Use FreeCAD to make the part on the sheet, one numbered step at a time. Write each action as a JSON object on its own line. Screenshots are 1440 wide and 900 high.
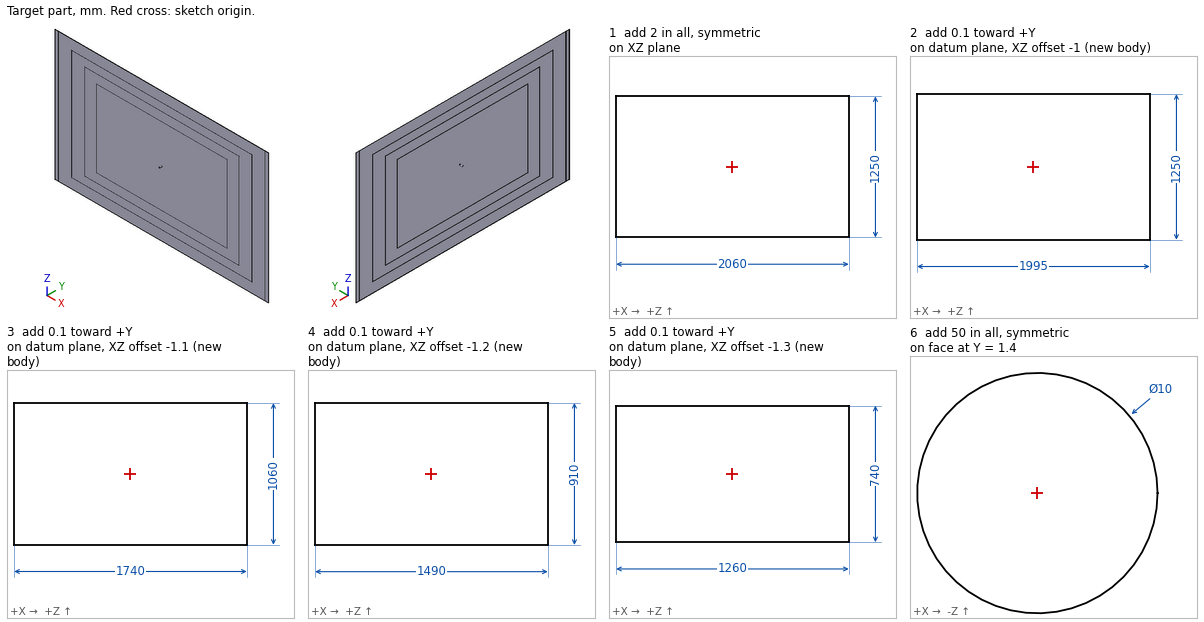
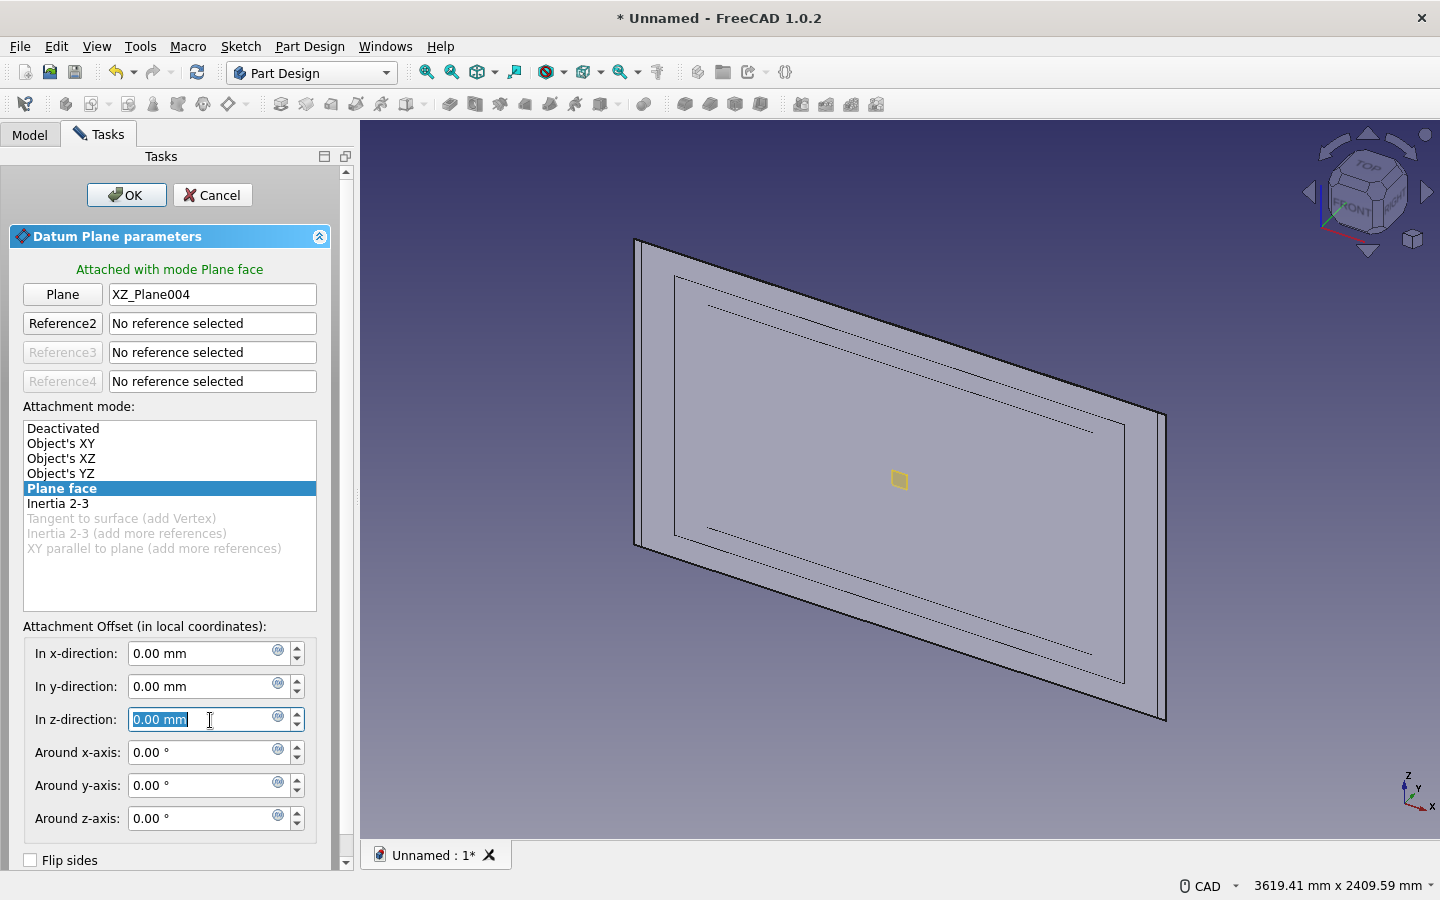
{"action": "type", "text": "-1.3"}
{"action": "key", "text": "Tab"}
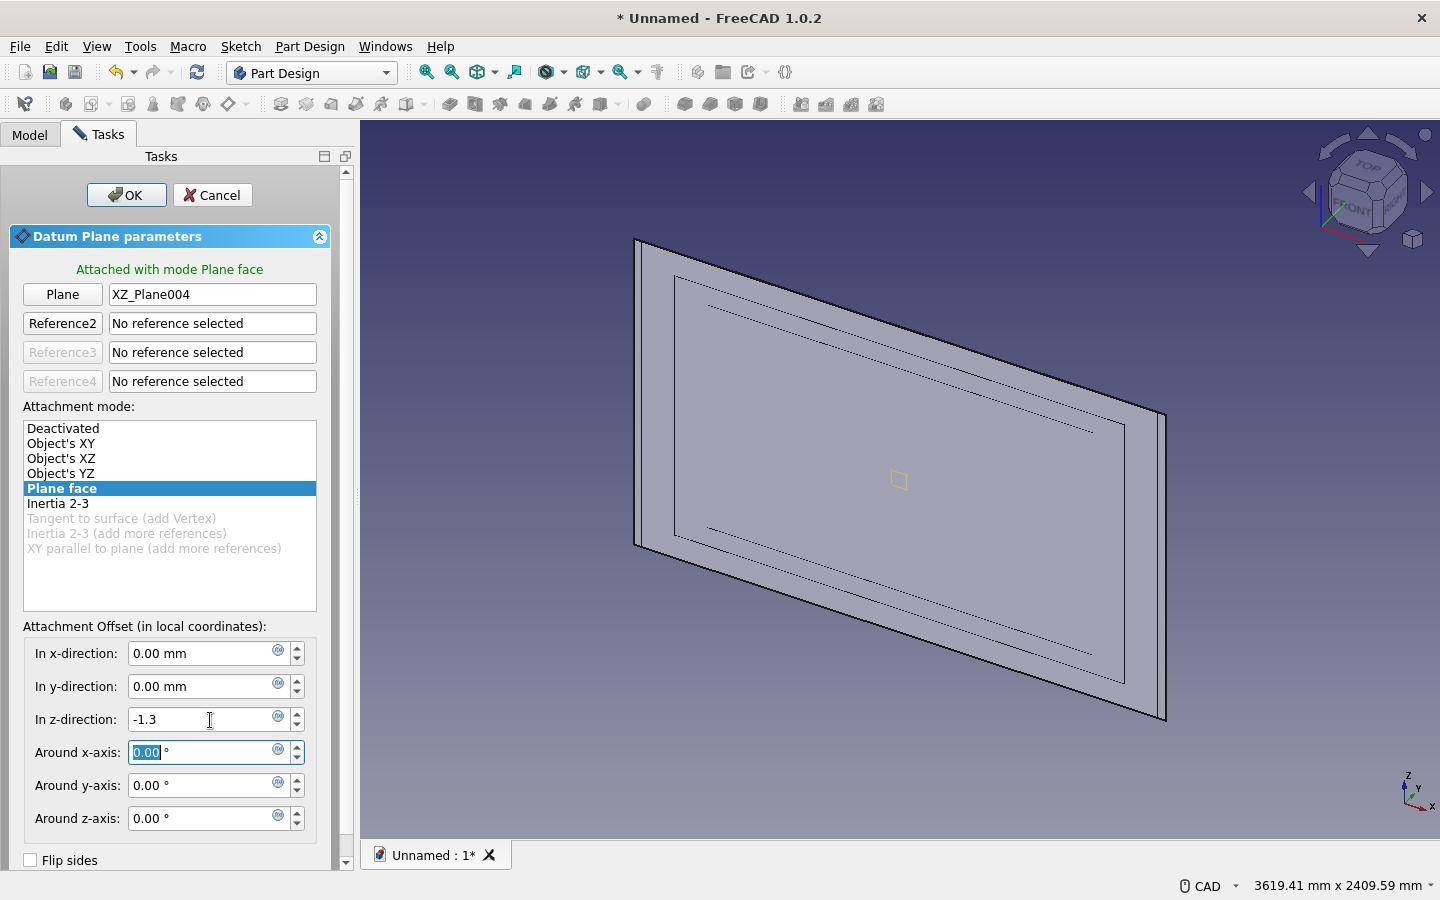
{"action": "left_click", "coordinate": [127, 195]}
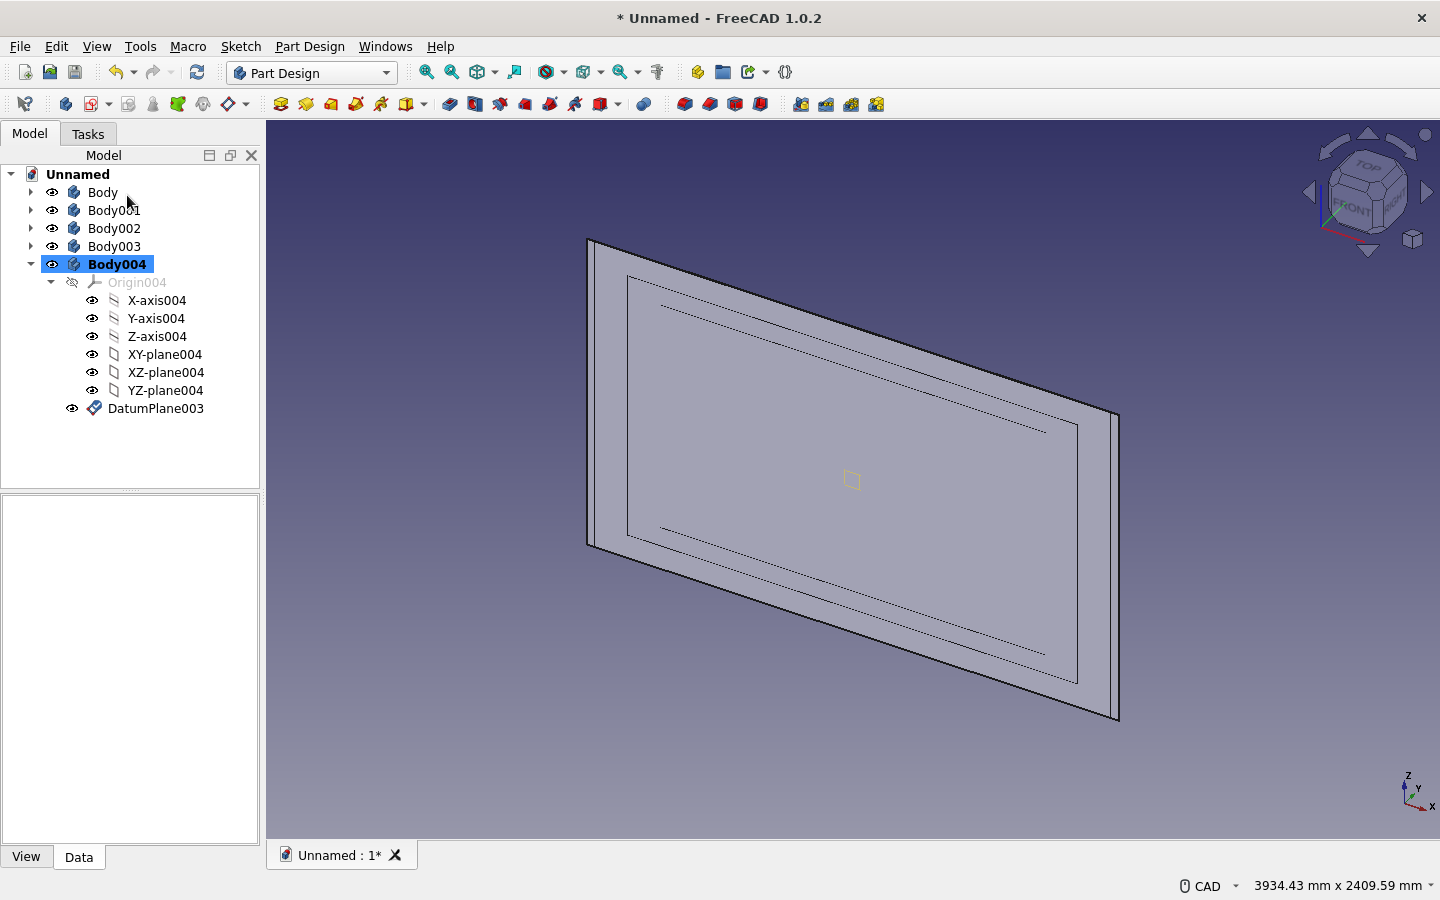
{"action": "left_click", "coordinate": [117, 408]}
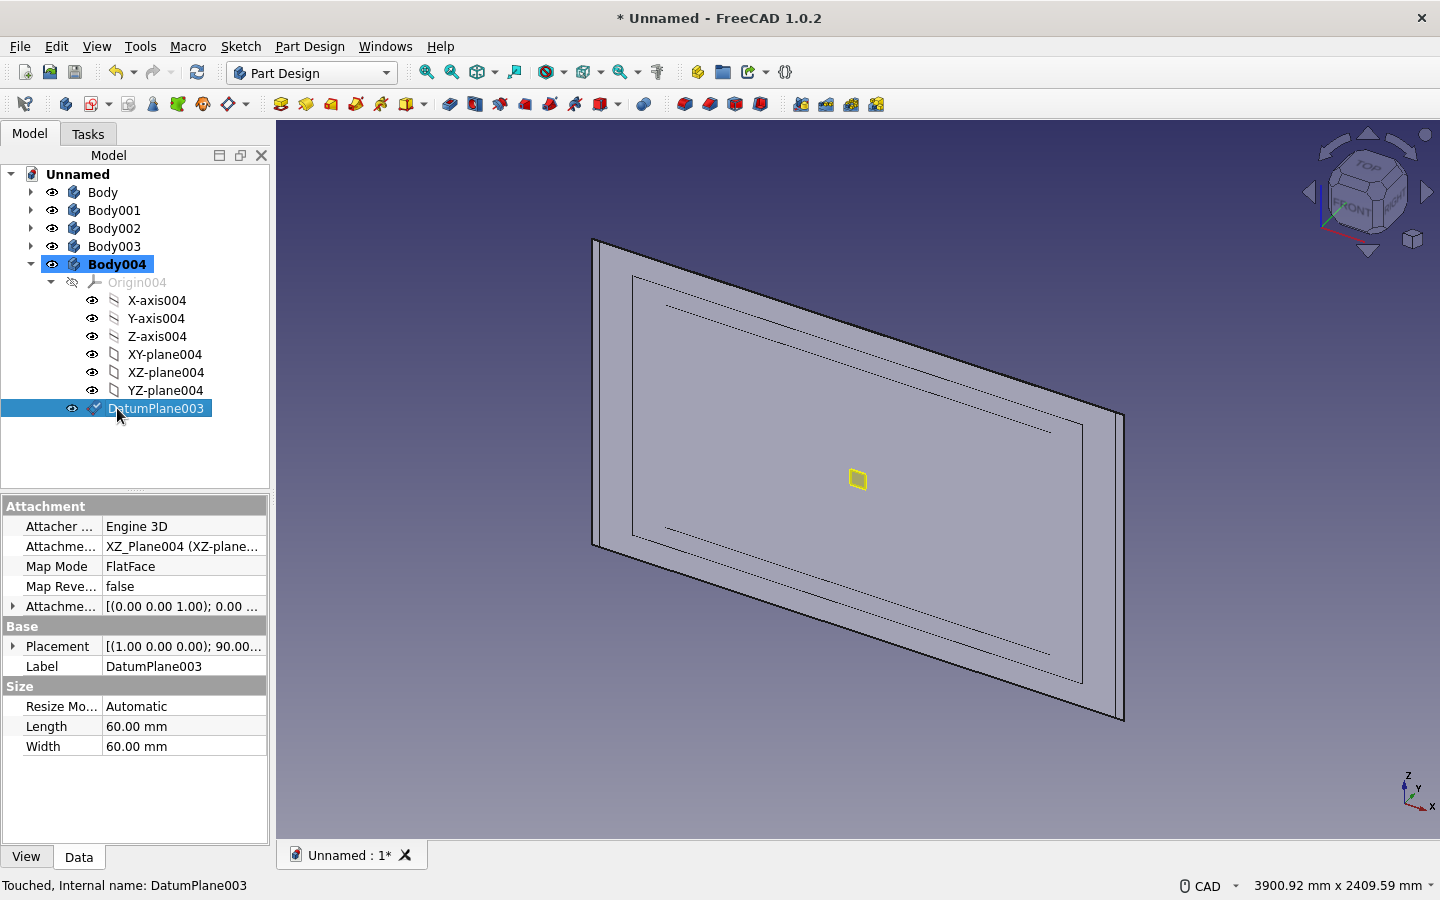
{"action": "left_click", "coordinate": [90, 104]}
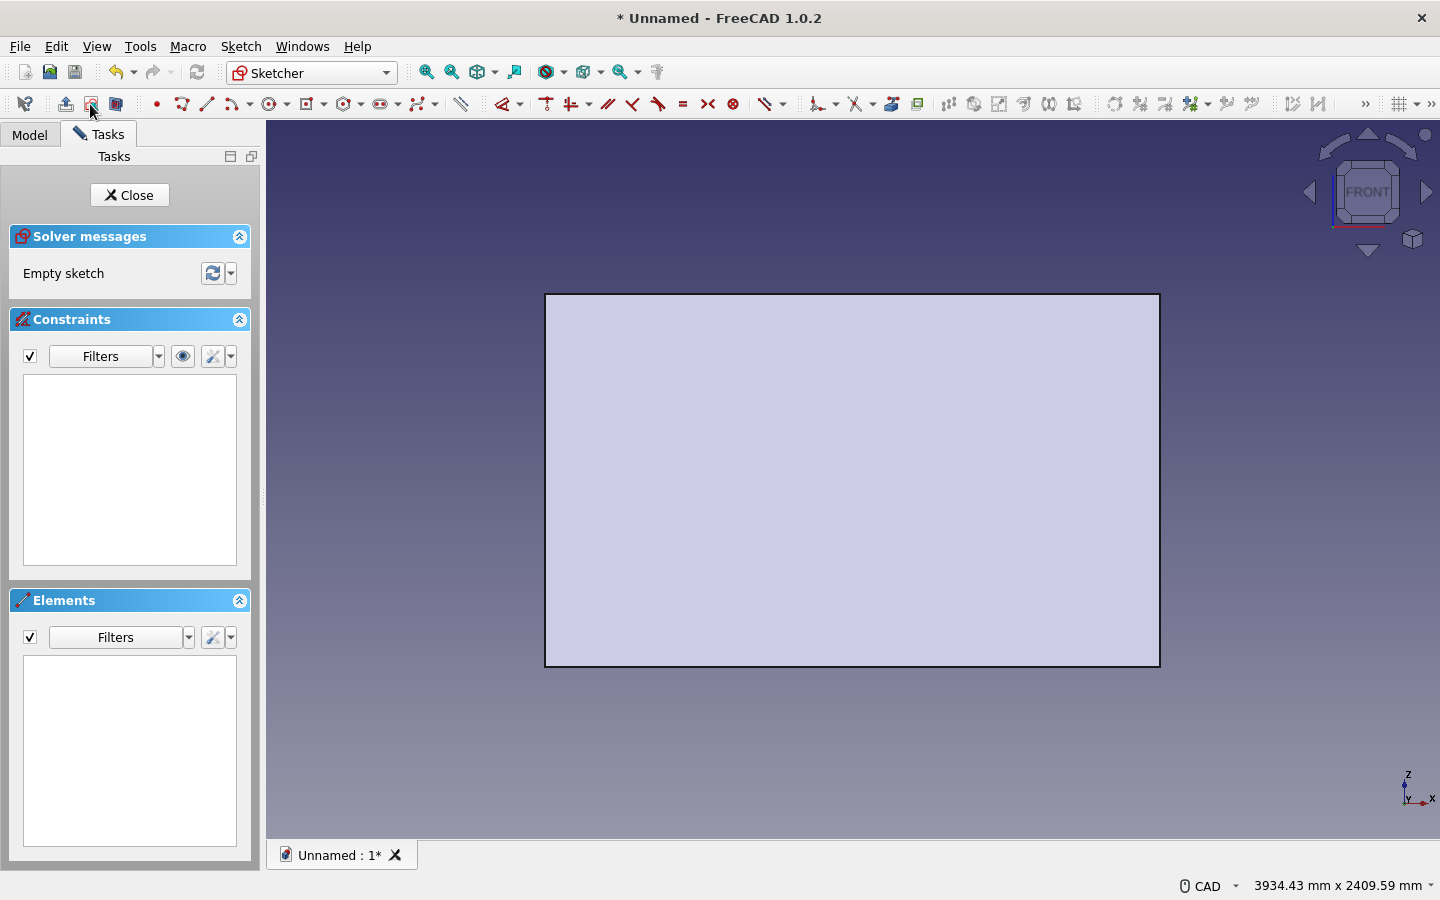
{"action": "scroll", "coordinate": [935, 481], "scroll_direction": "up", "scroll_amount": 3}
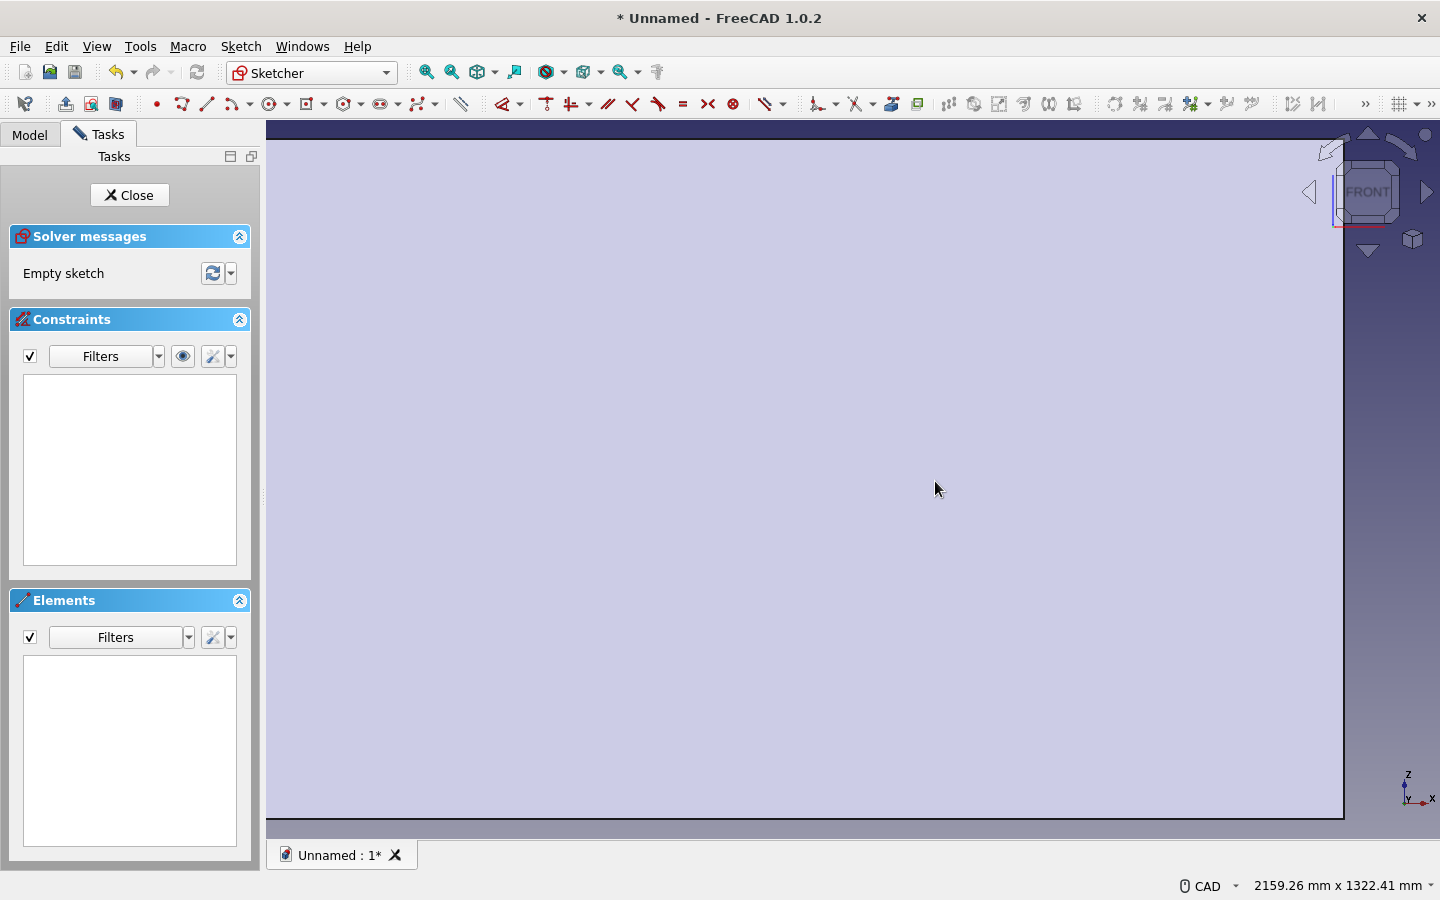
{"action": "left_click", "coordinate": [306, 104]}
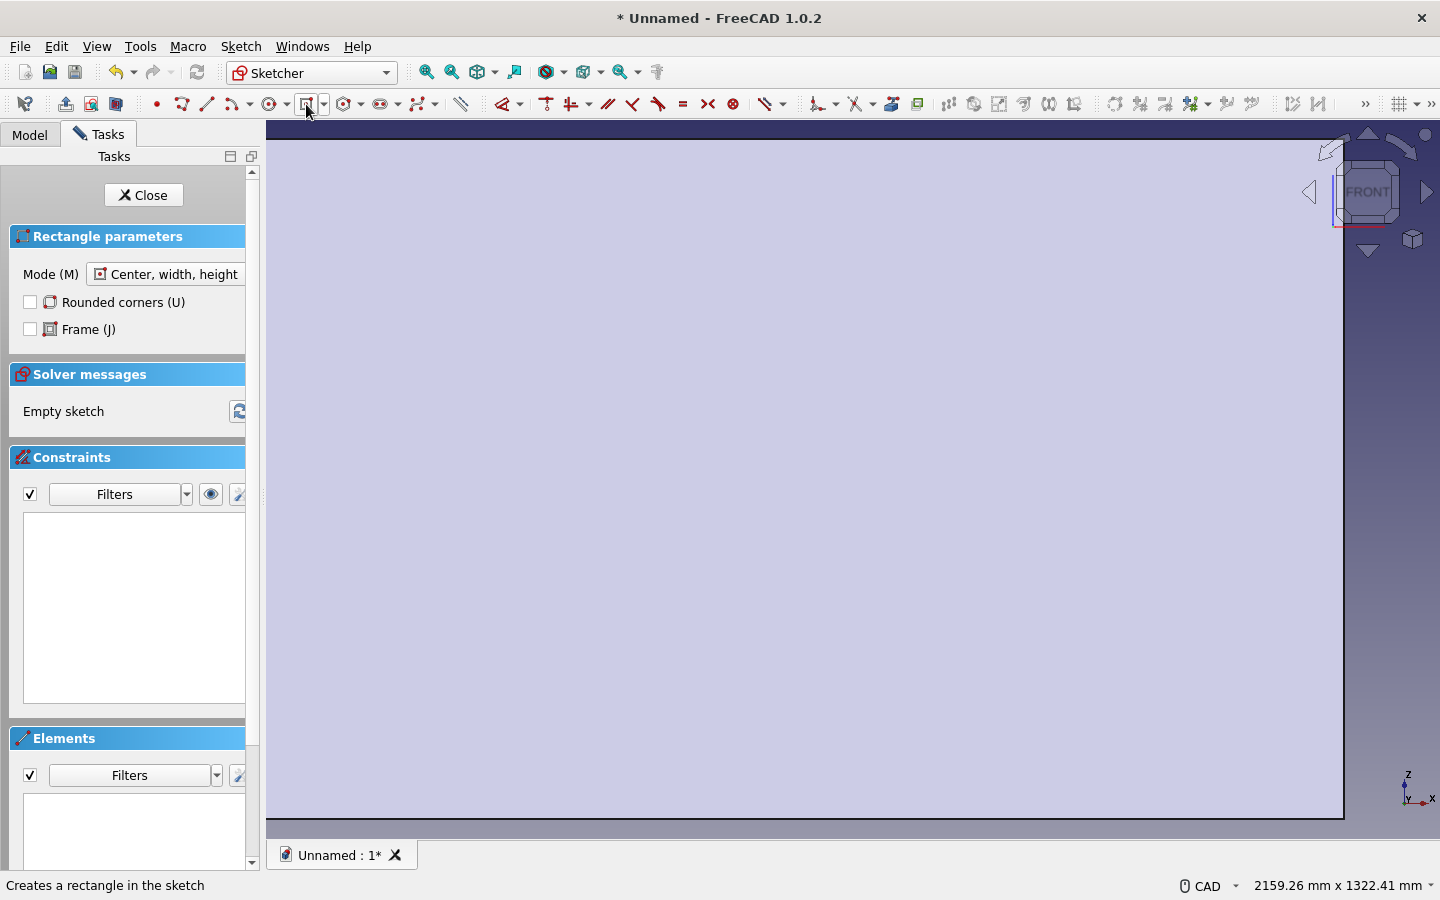
{"action": "left_click", "coordinate": [784, 479]}
{"action": "mouse_move", "coordinate": [1127, 278]}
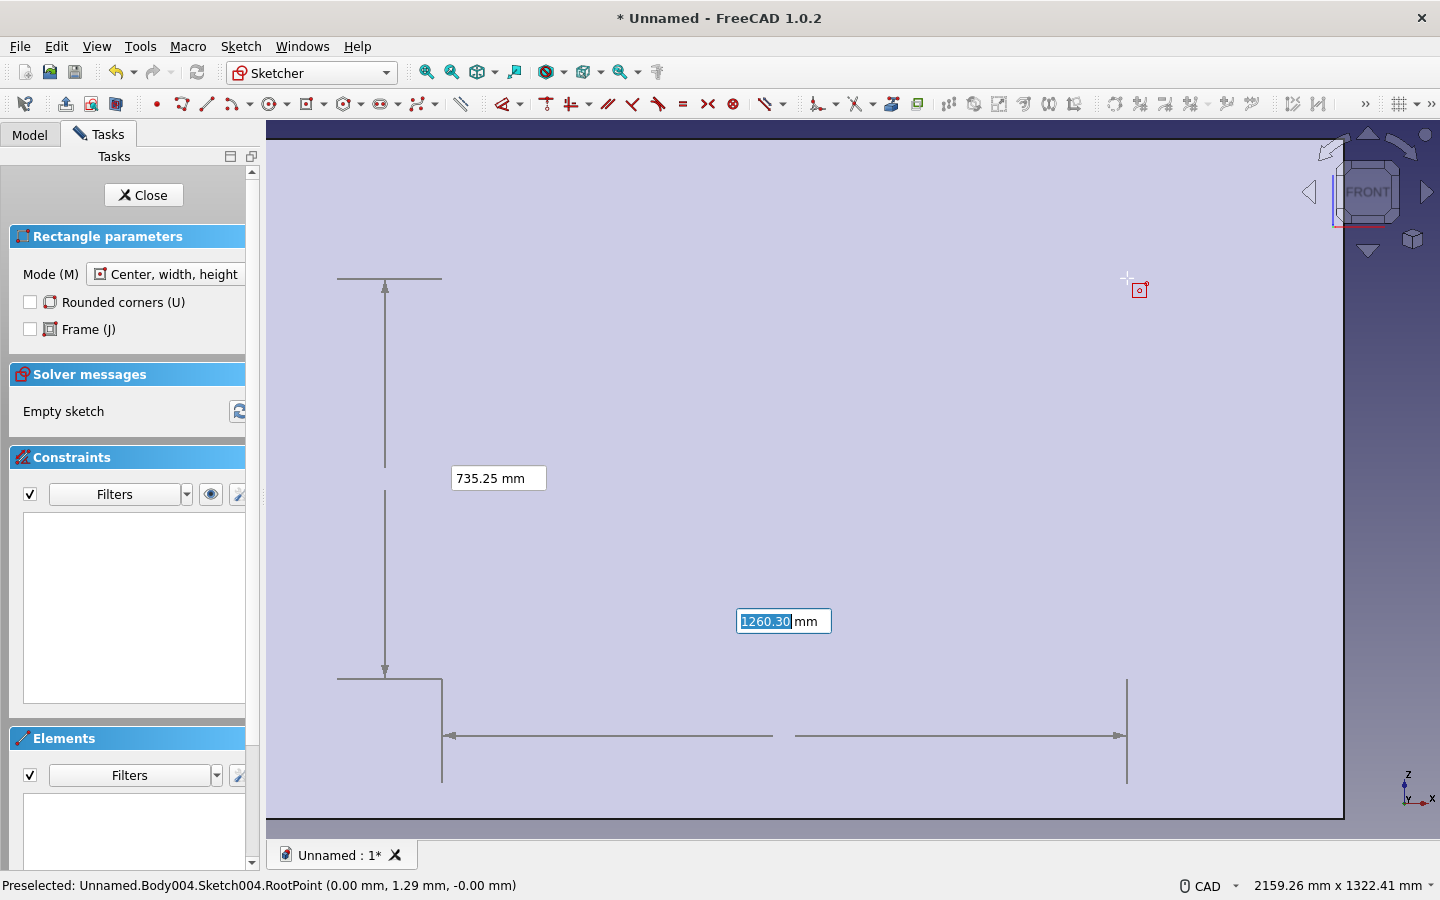
{"action": "type", "text": "1260"}
{"action": "key", "text": "Tab"}
{"action": "type", "text": "740"}
{"action": "key", "text": "Return"}
{"action": "key", "text": "Escape"}